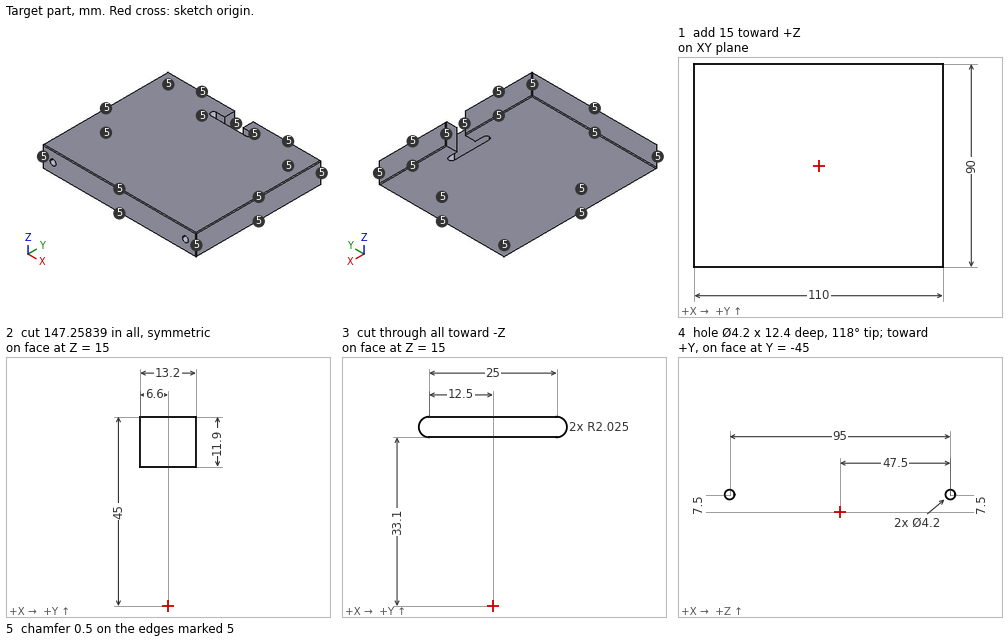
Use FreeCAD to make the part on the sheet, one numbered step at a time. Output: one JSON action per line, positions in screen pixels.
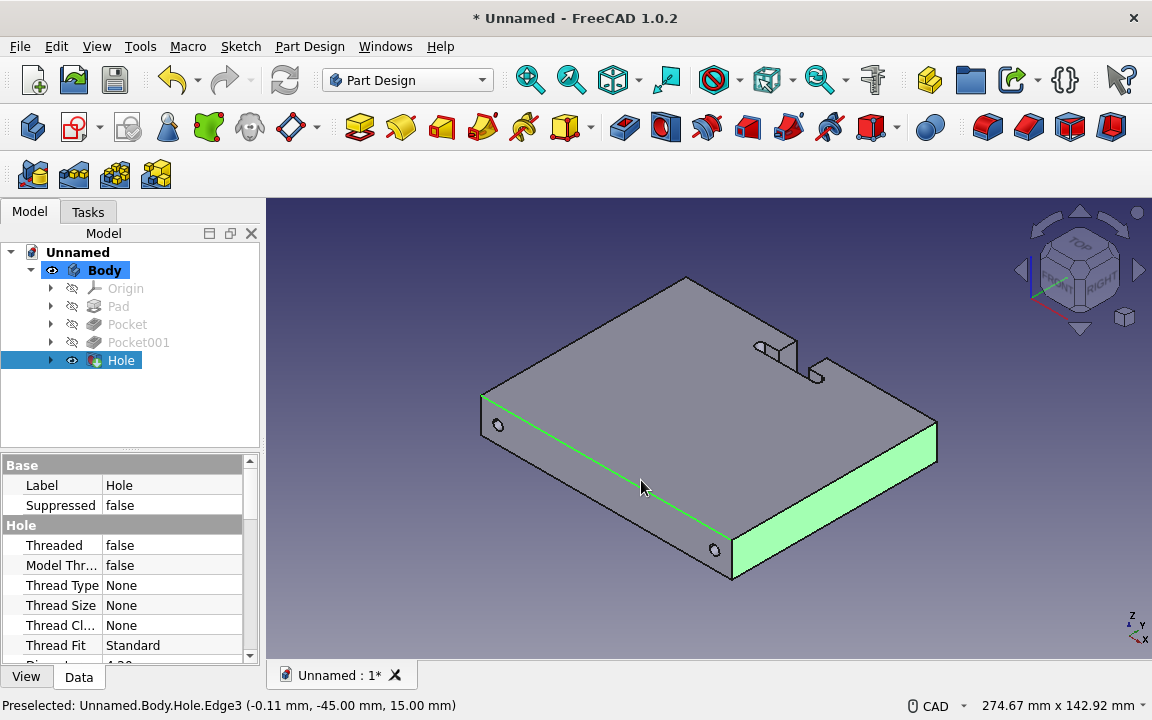
{"action": "key", "text": "2"}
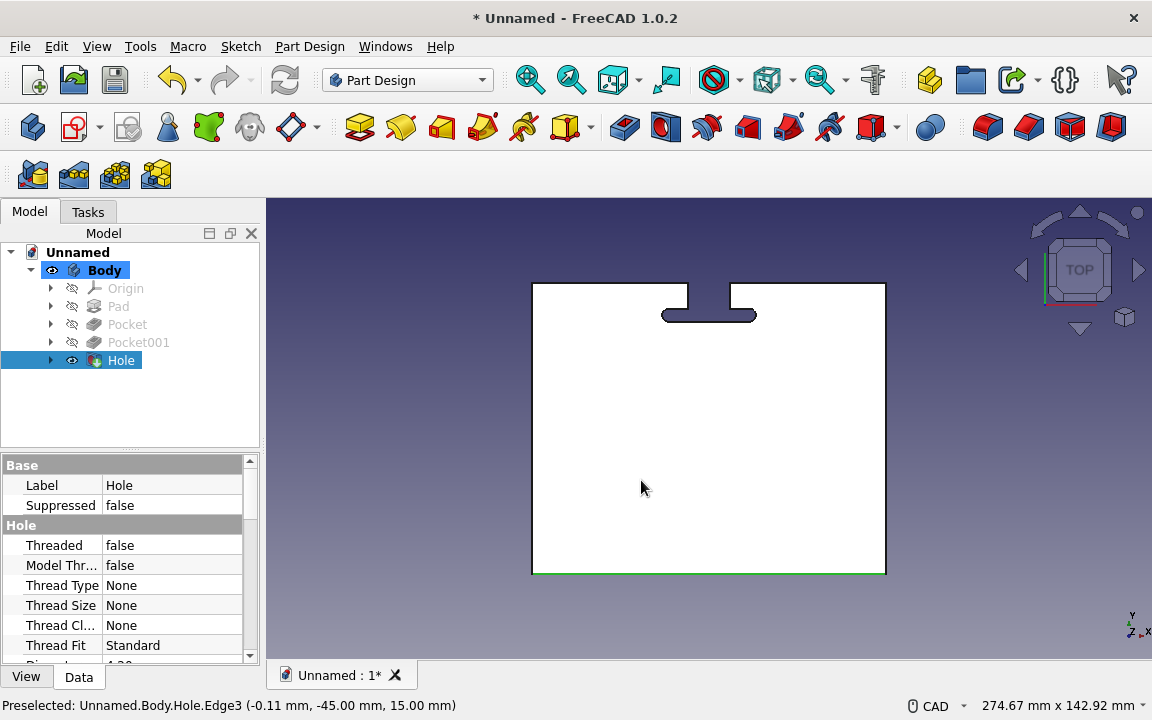
{"action": "key", "text": "1"}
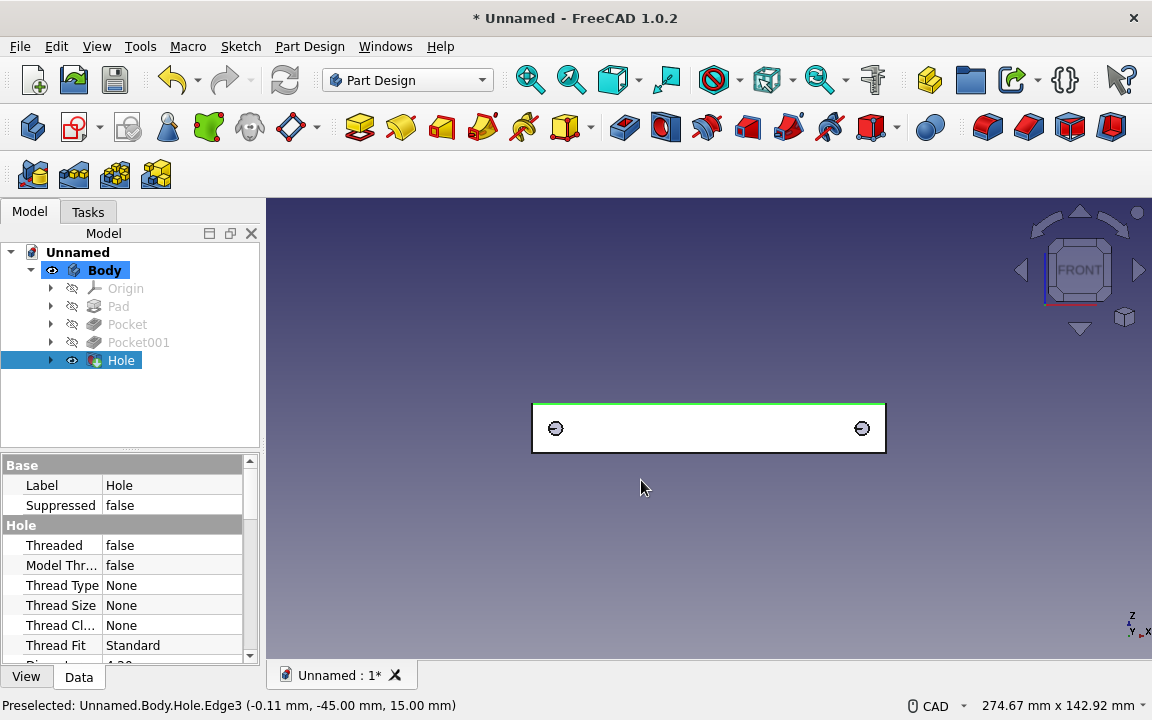
{"action": "key", "text": "v f"}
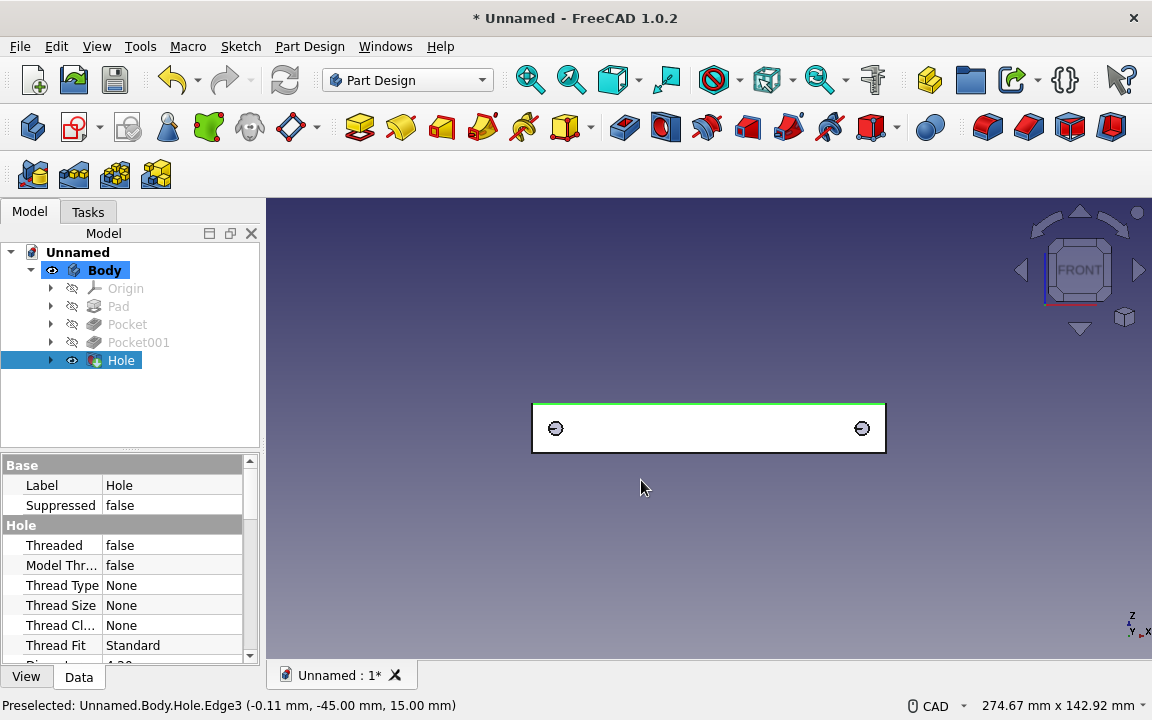
{"action": "left_click", "coordinate": [709, 452], "text": "ctrl"}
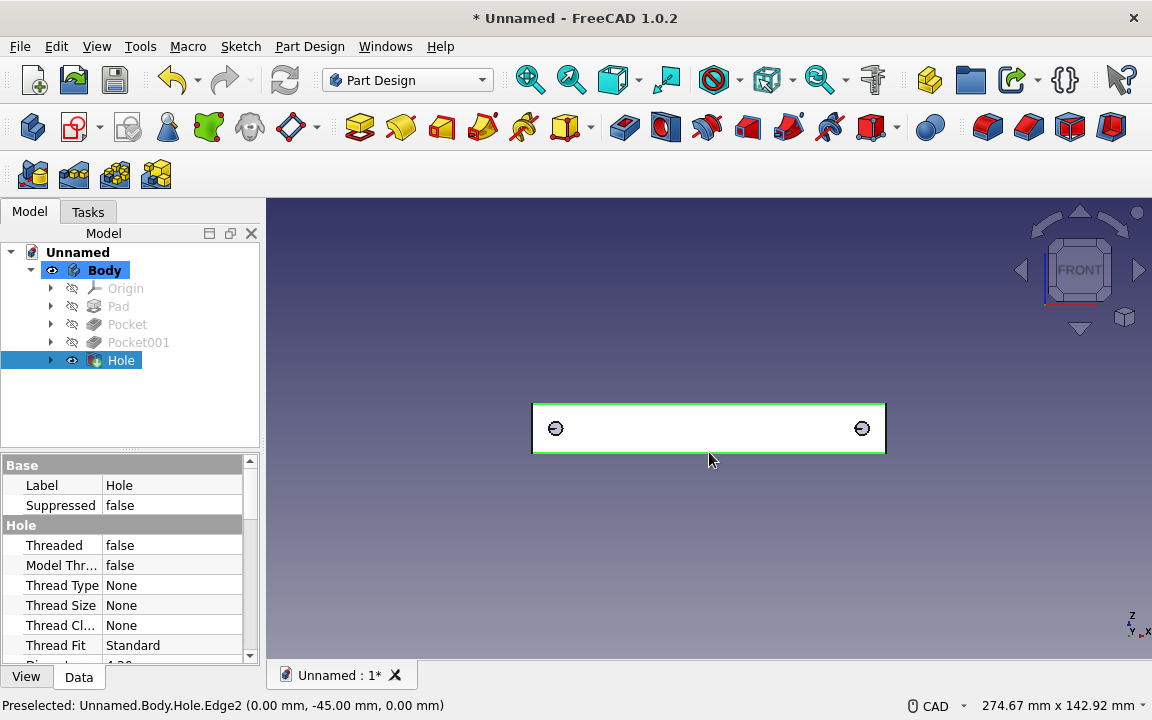
{"action": "key", "text": "3"}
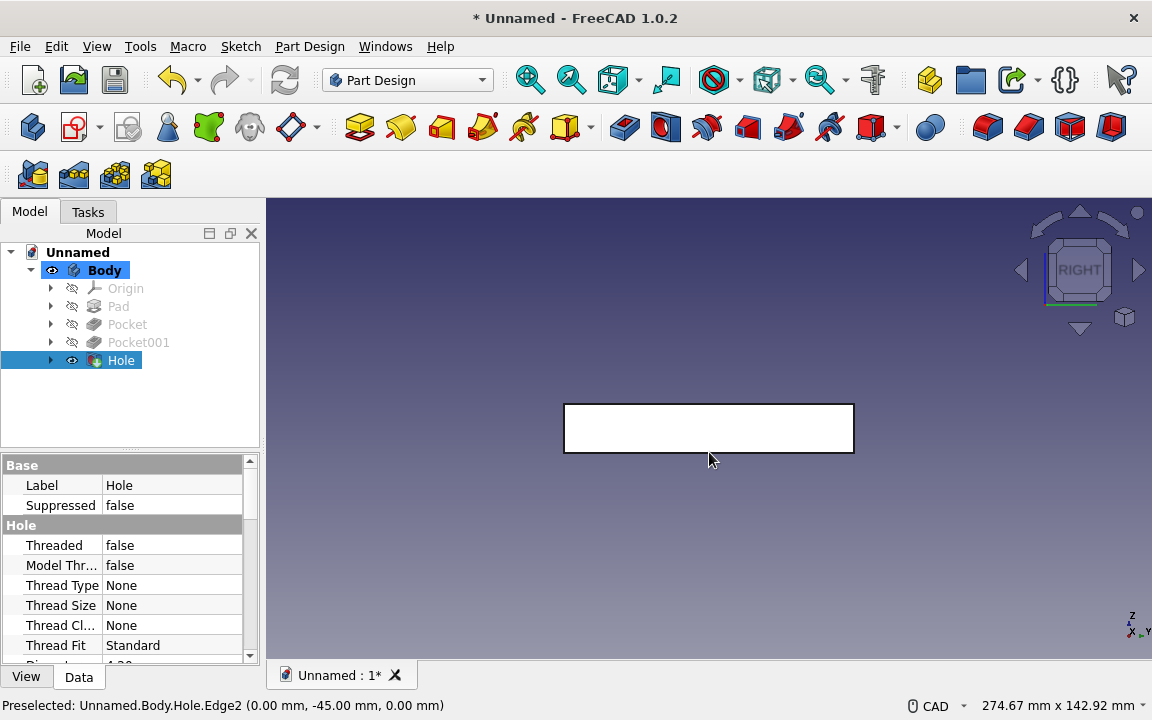
{"action": "left_click", "coordinate": [531, 80]}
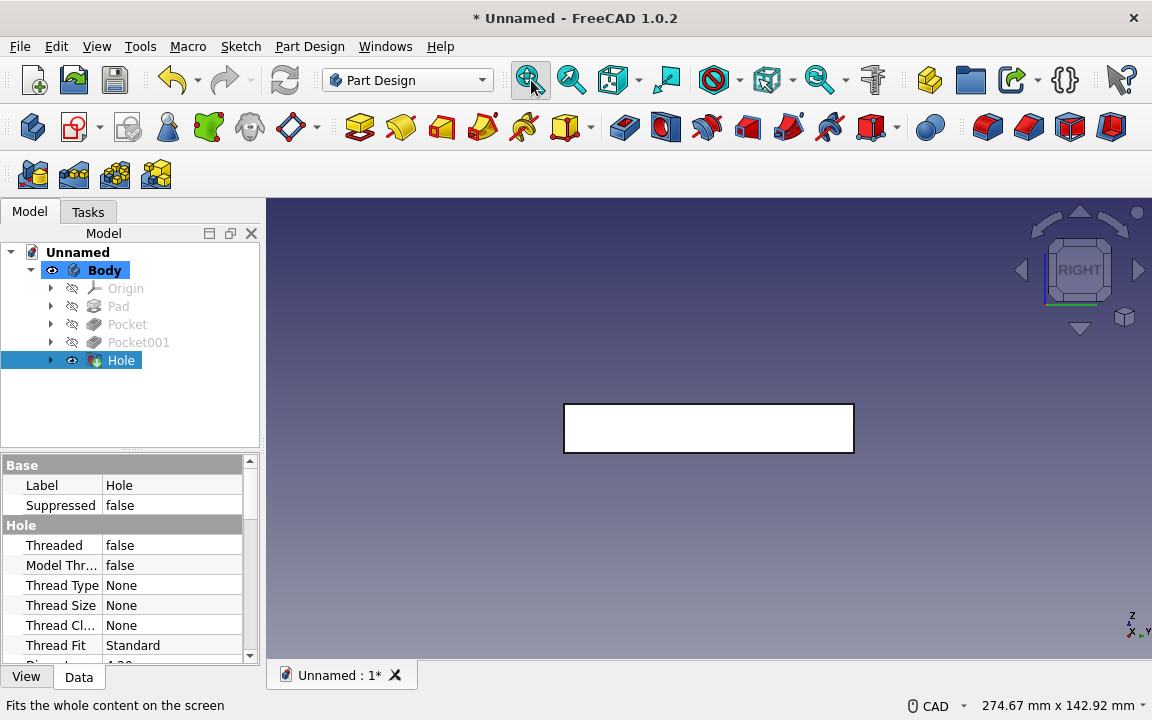
{"action": "key", "text": "5"}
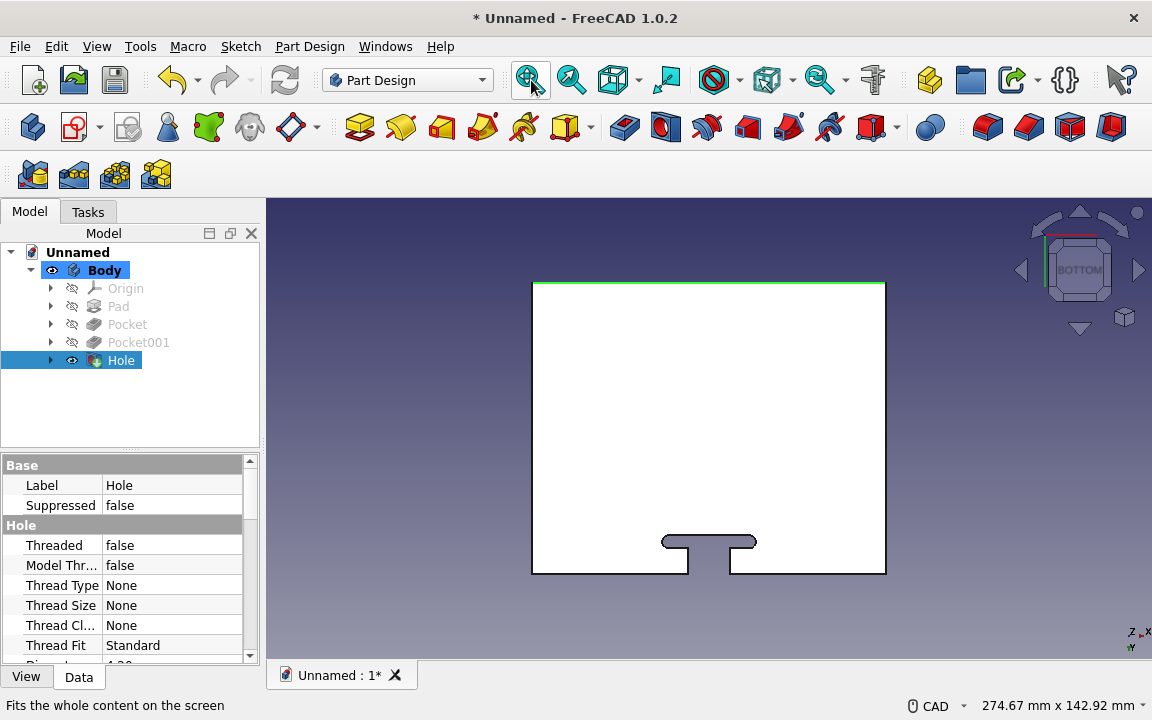
{"action": "key", "text": "4"}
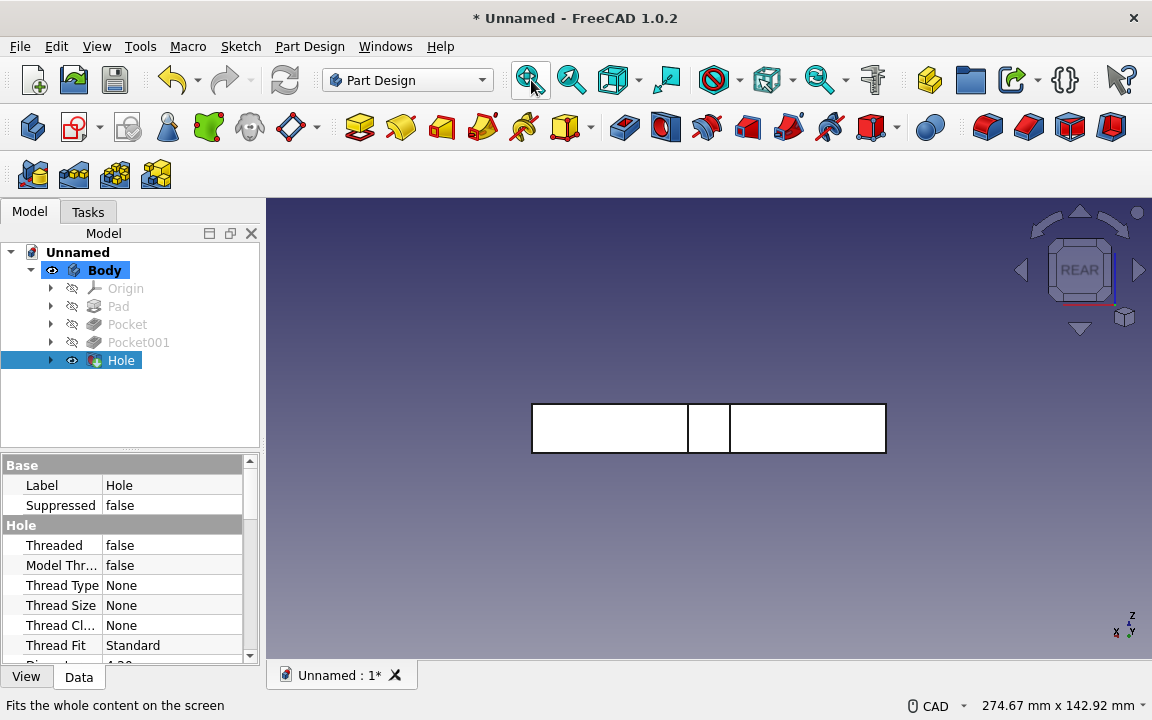
{"action": "left_click", "coordinate": [531, 80]}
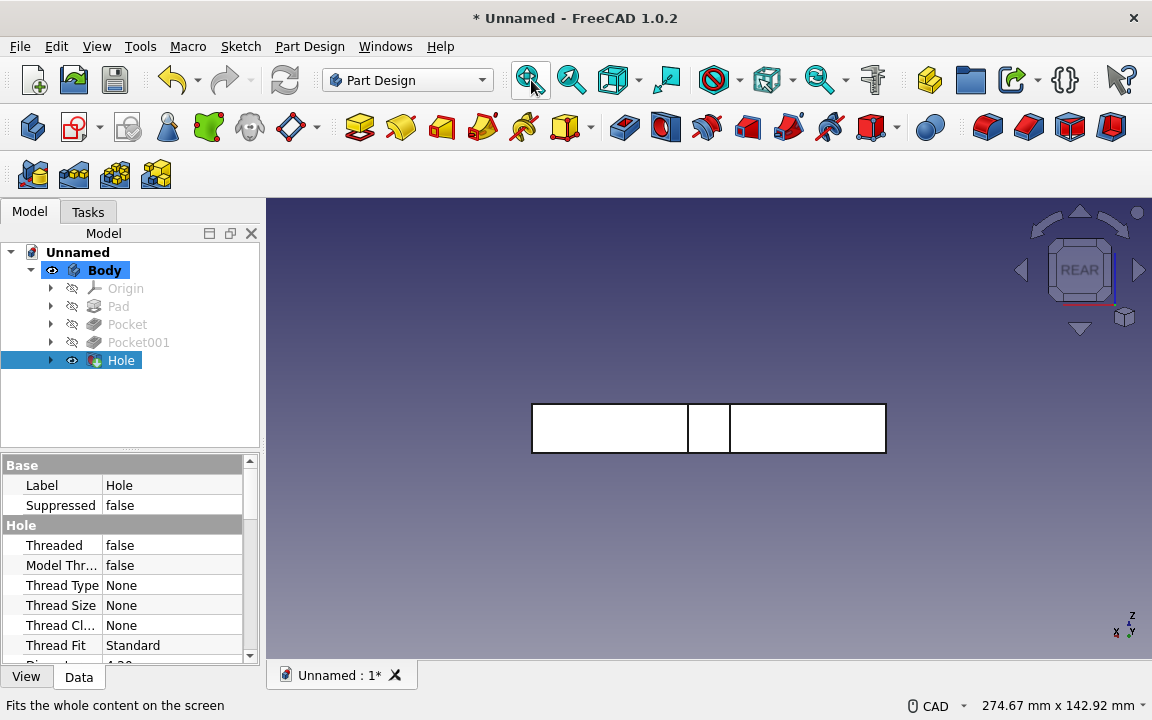
{"action": "left_click", "coordinate": [764, 428], "text": "ctrl"}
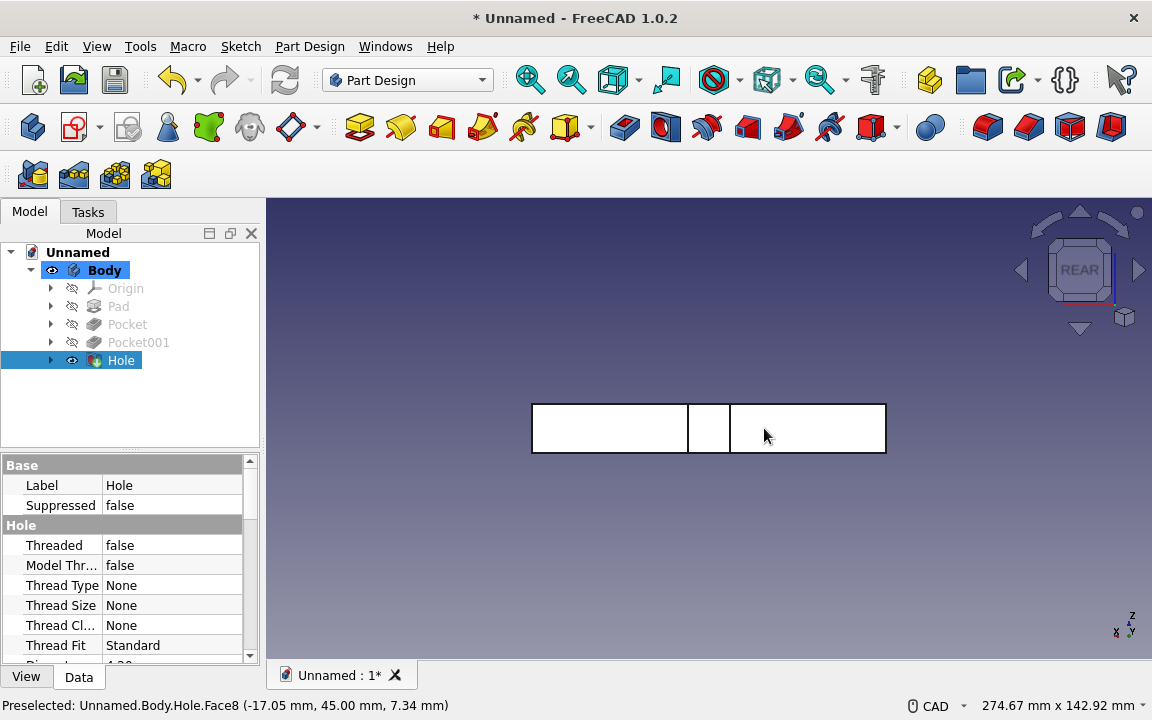
{"action": "left_click", "coordinate": [565, 428], "text": "ctrl"}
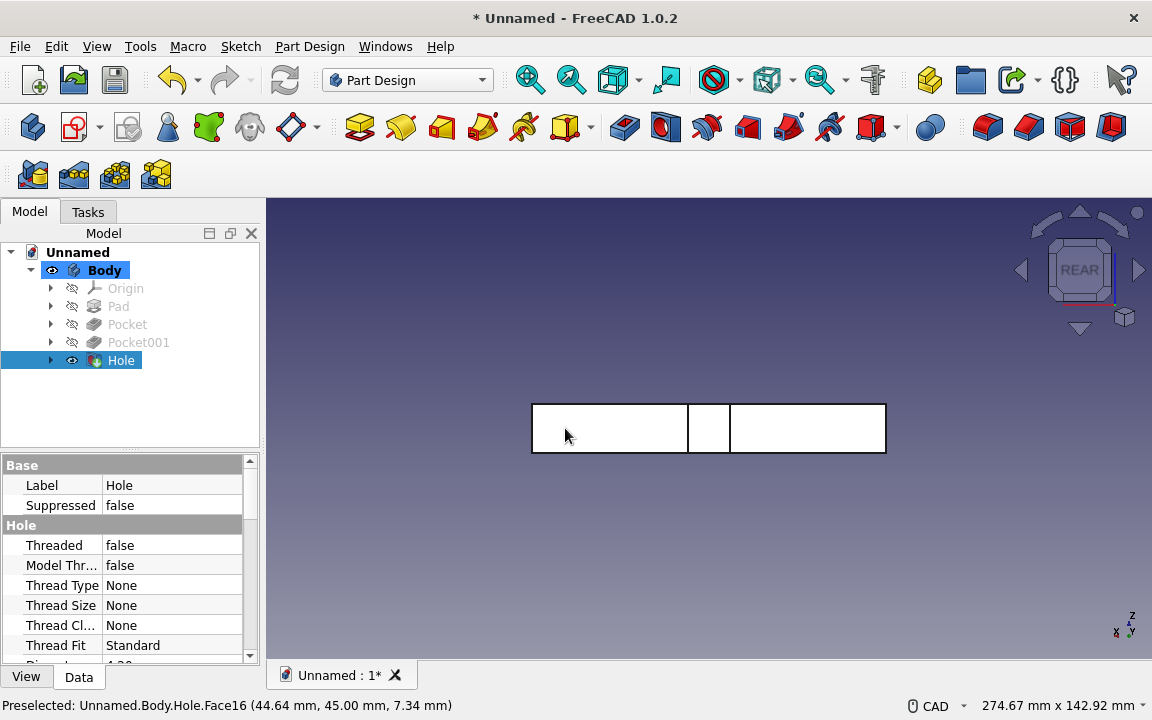
{"action": "key", "text": "6"}